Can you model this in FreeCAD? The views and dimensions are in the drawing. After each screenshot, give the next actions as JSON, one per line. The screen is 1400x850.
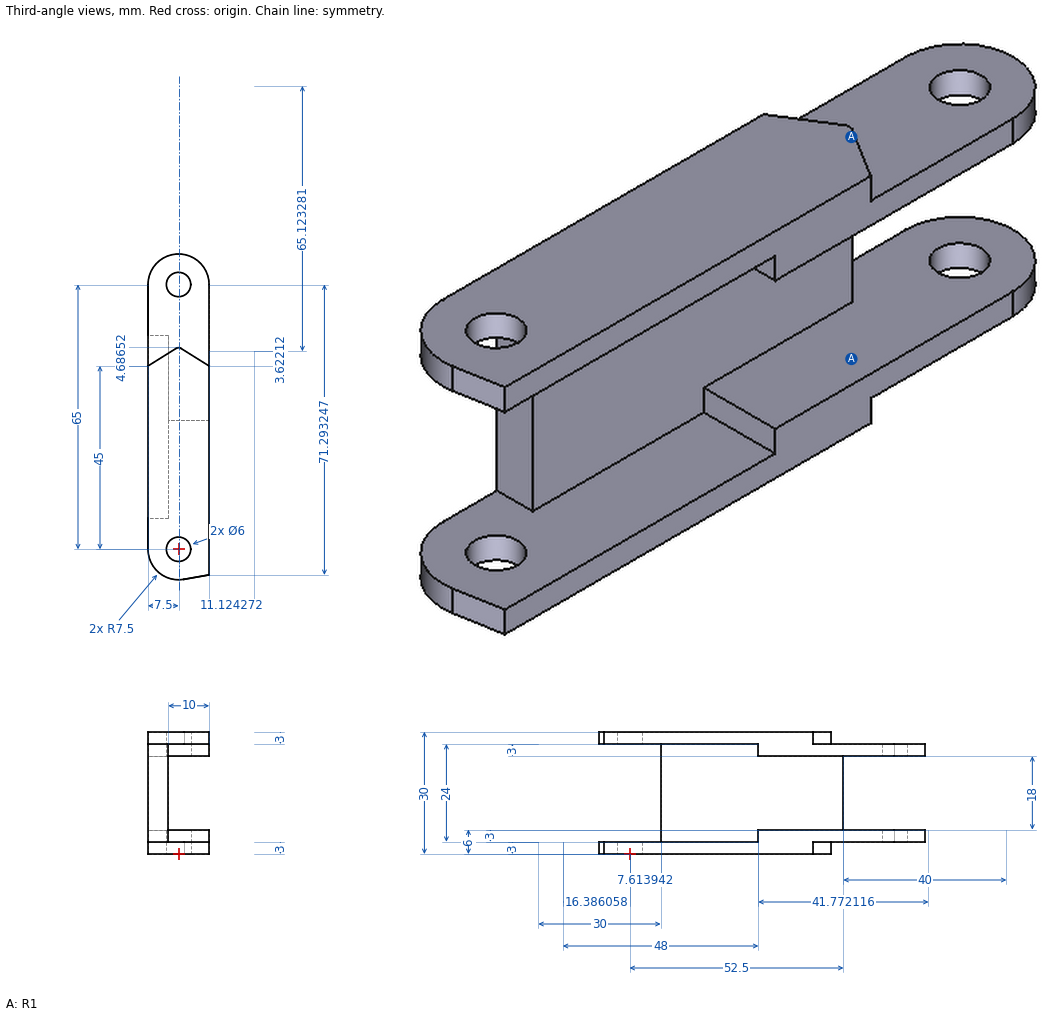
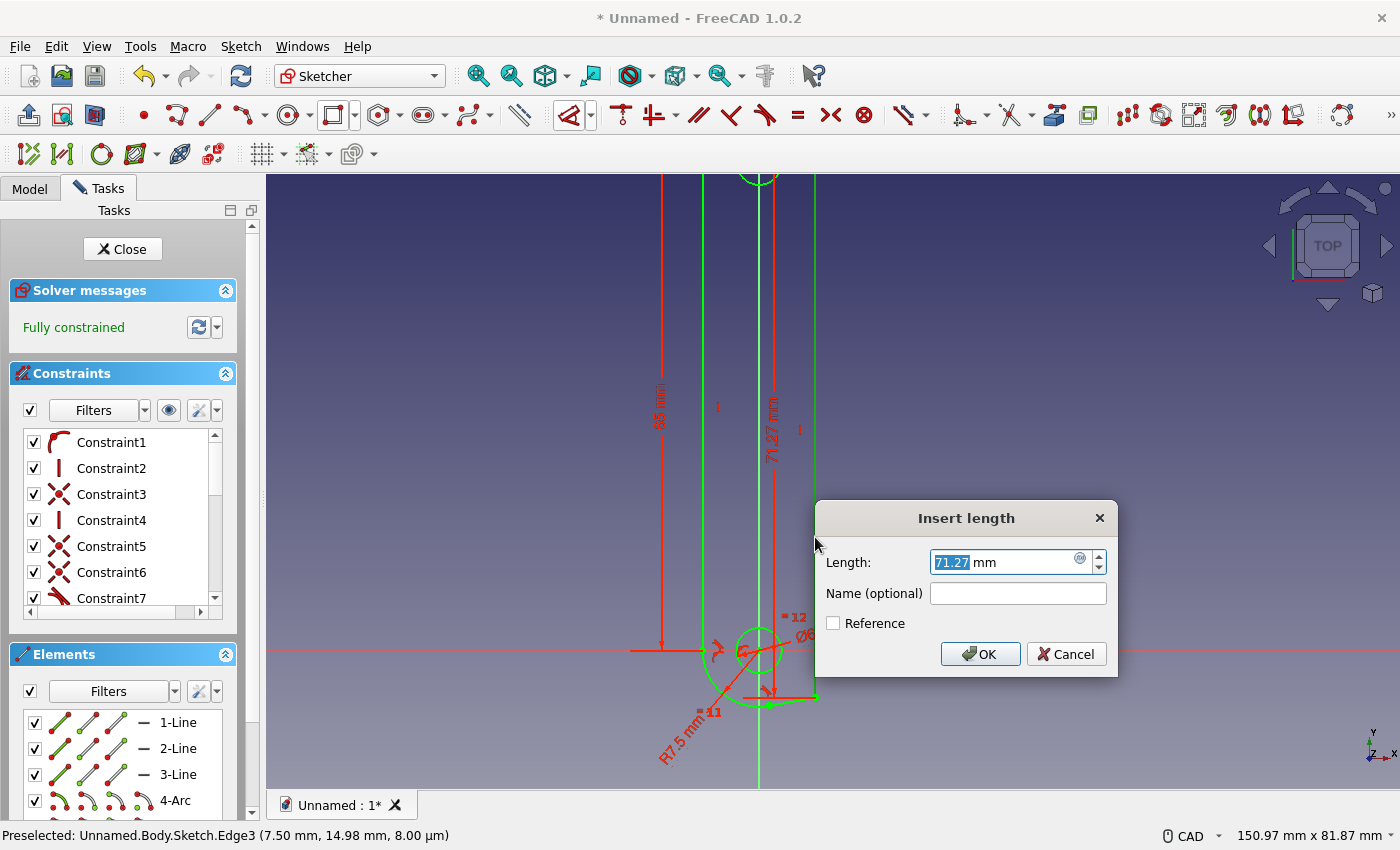
{"action": "type", "text": "71.293247"}
{"action": "key", "text": "Return"}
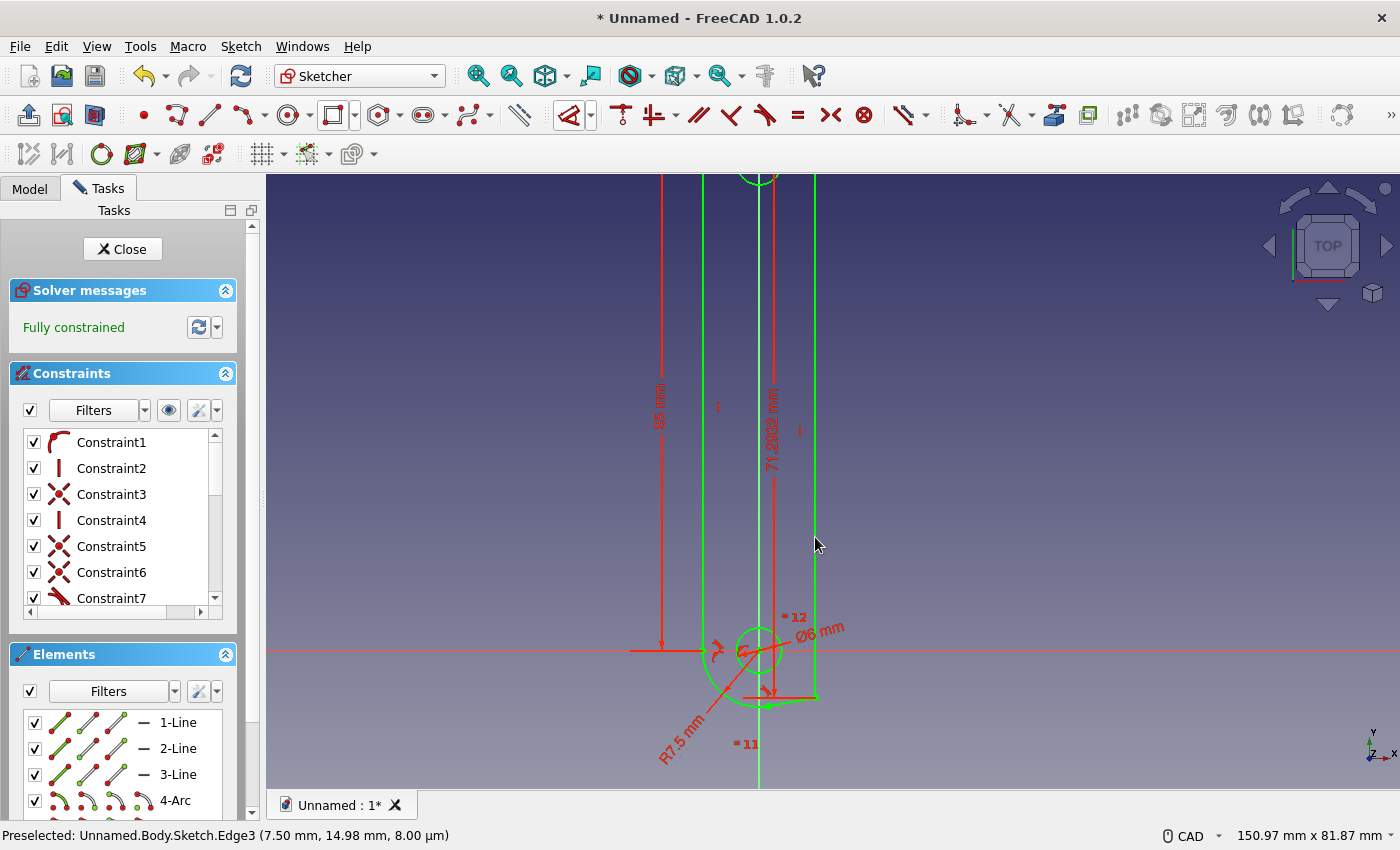
{"action": "left_click", "coordinate": [123, 249]}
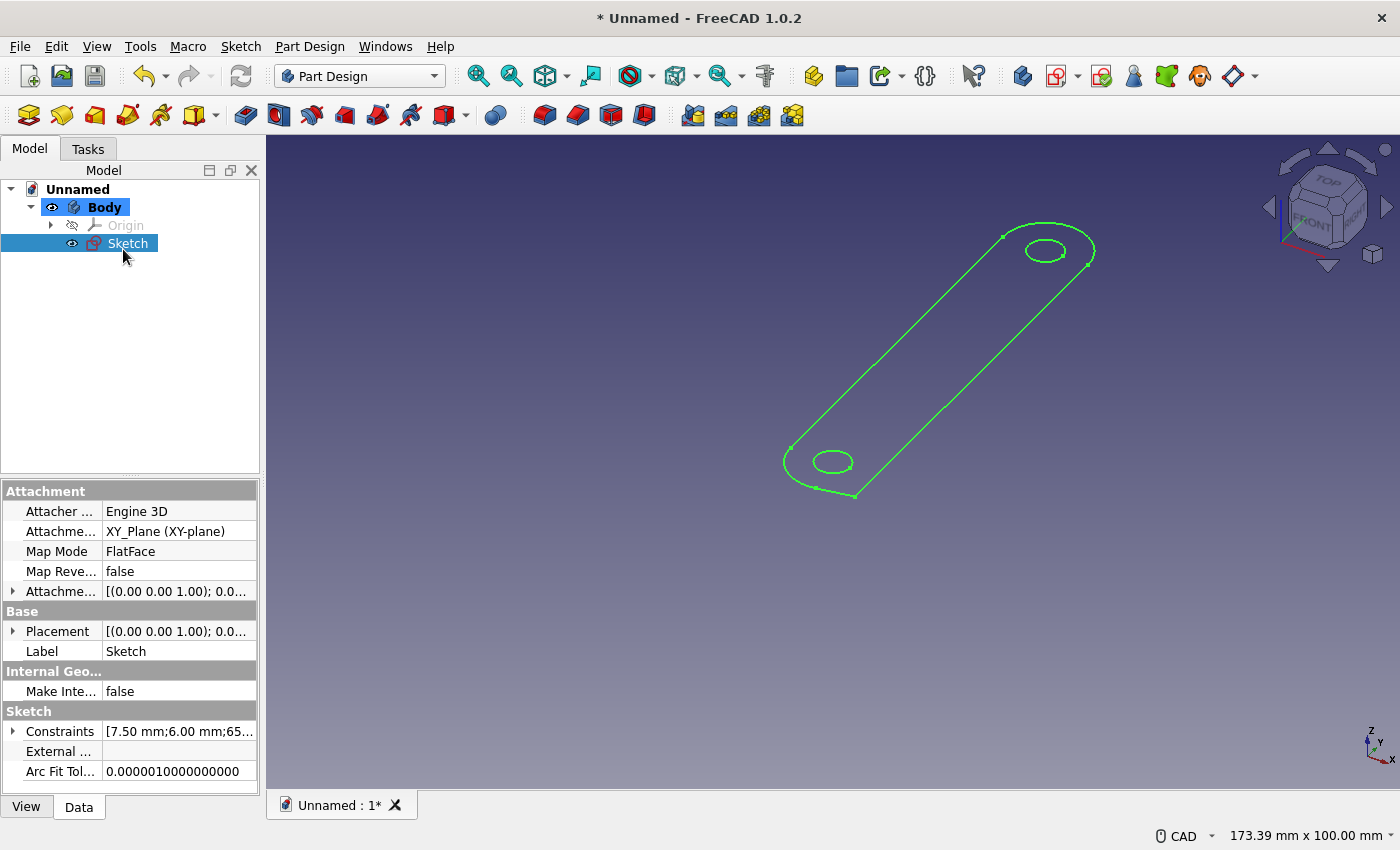
{"action": "left_click", "coordinate": [29, 116]}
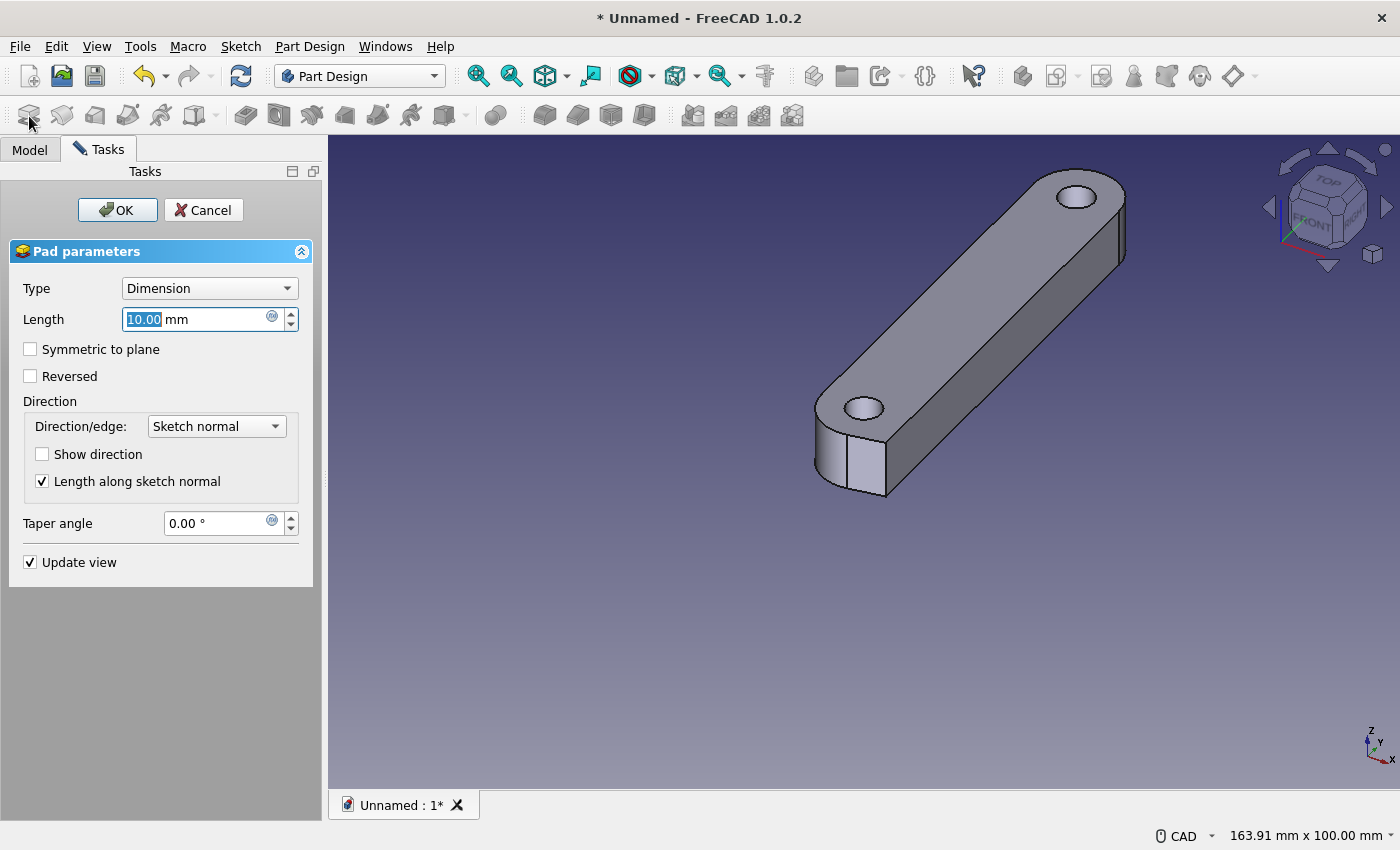
{"action": "type", "text": "30"}
{"action": "key", "text": "Tab"}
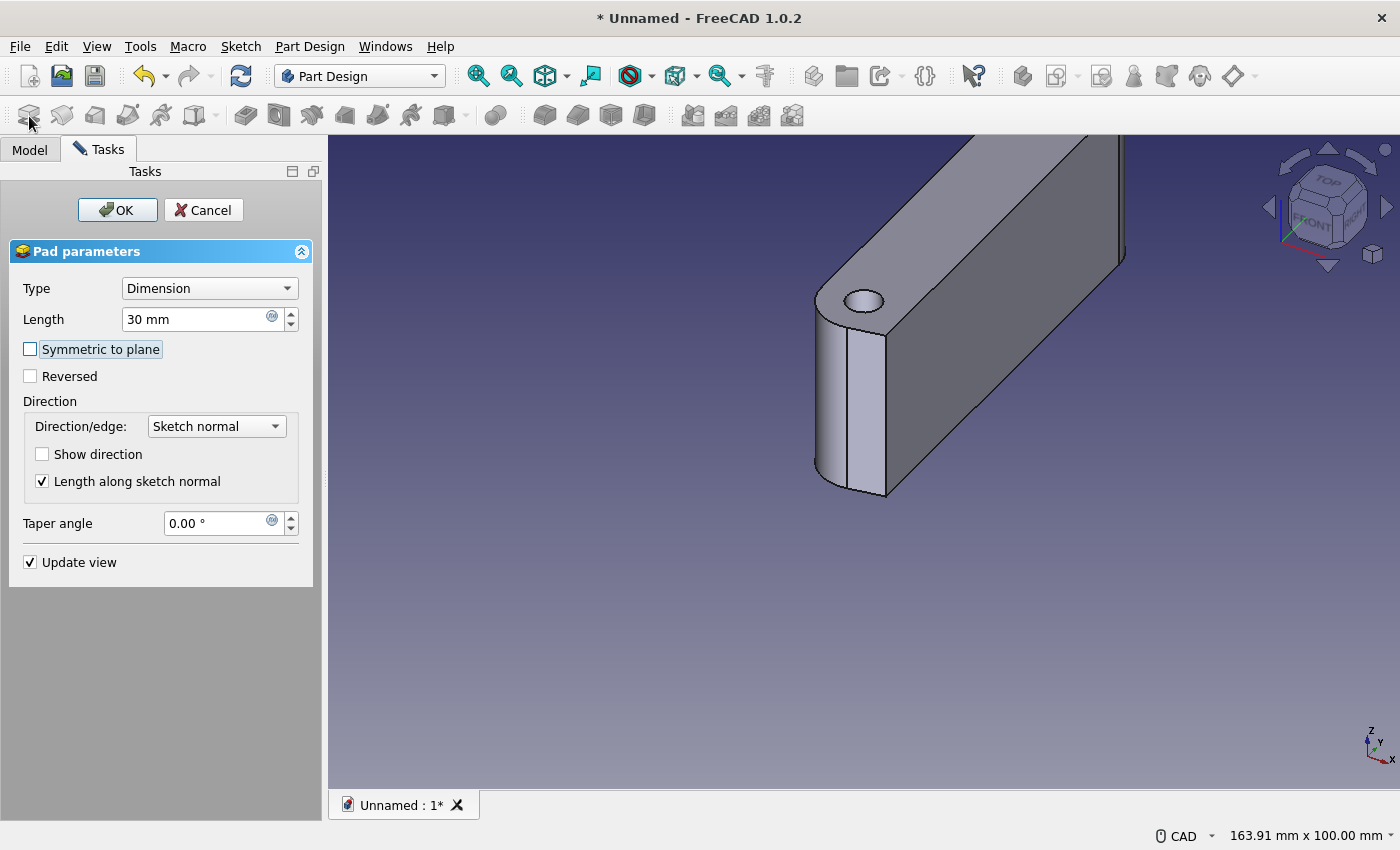
{"action": "left_click", "coordinate": [118, 210]}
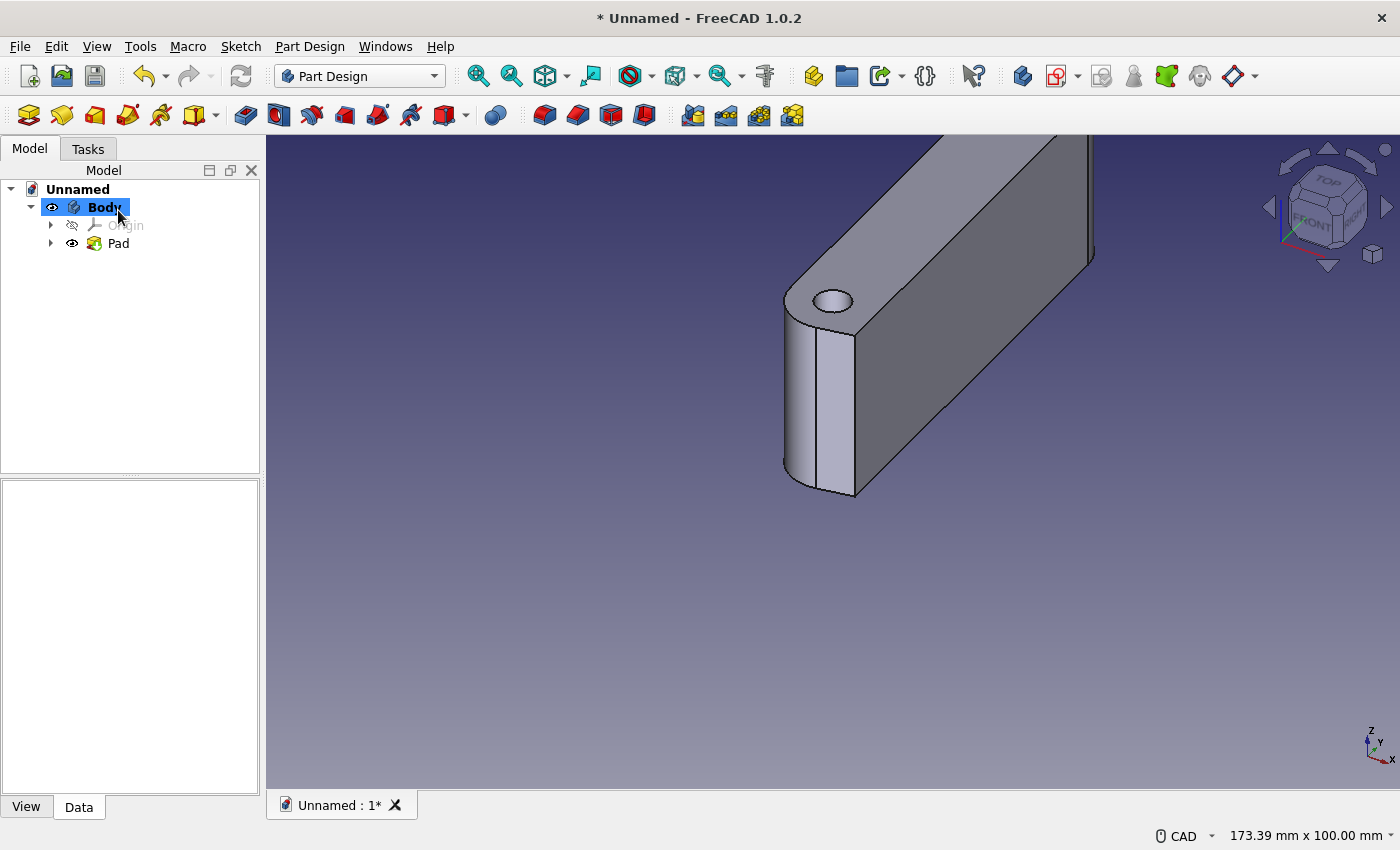
{"action": "key", "text": "v f"}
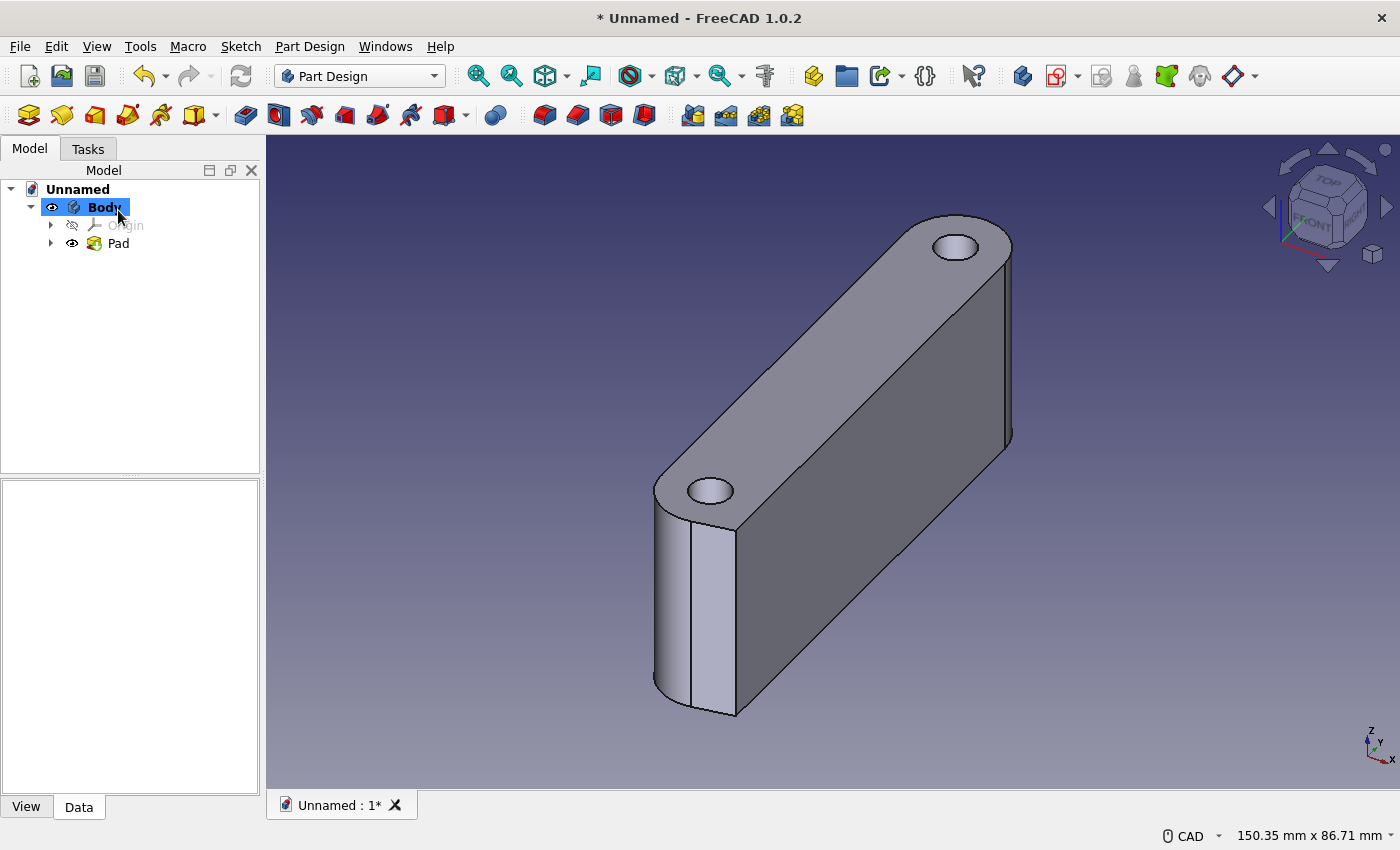
{"action": "left_click", "coordinate": [947, 413]}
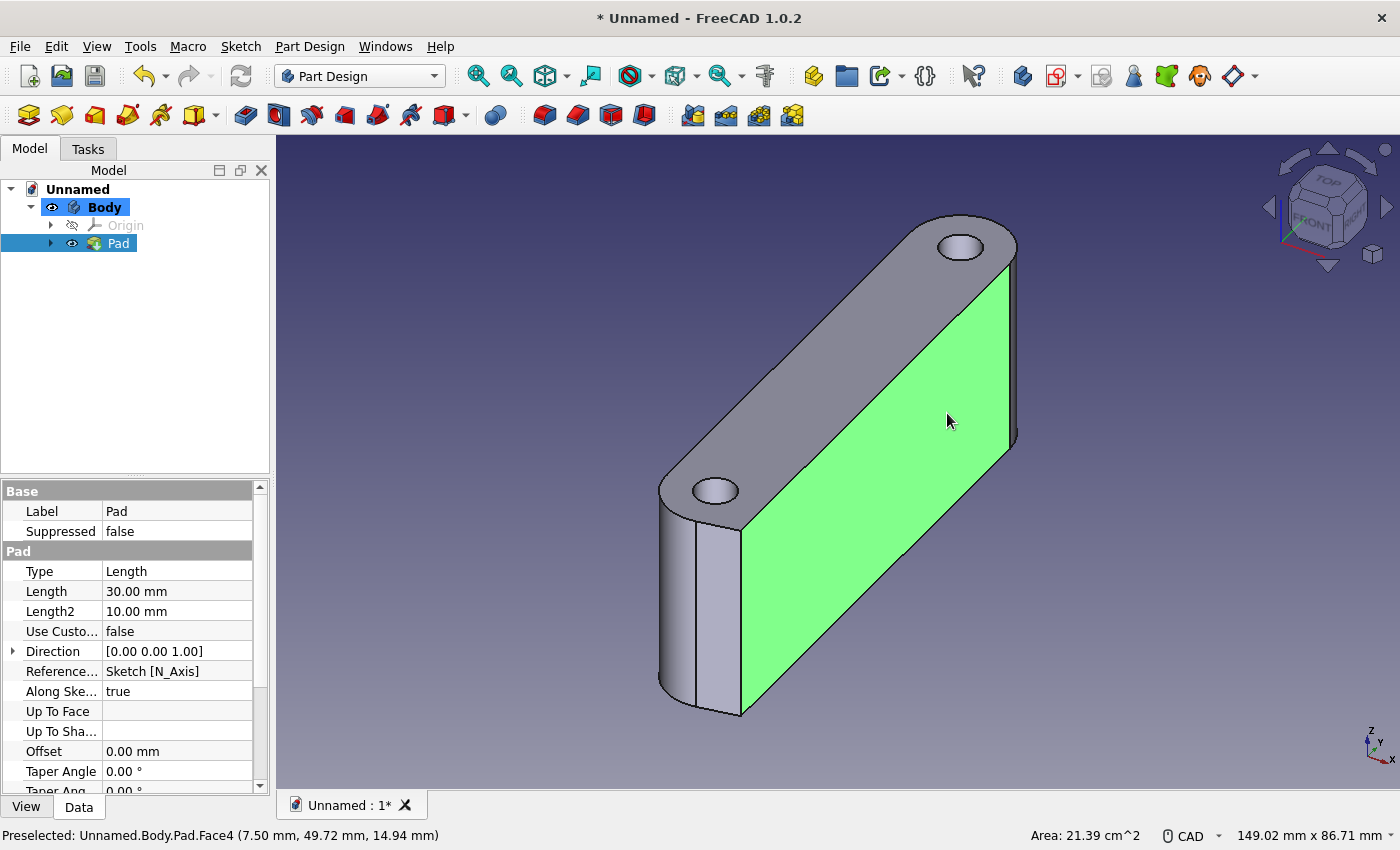
{"action": "left_click", "coordinate": [1056, 76]}